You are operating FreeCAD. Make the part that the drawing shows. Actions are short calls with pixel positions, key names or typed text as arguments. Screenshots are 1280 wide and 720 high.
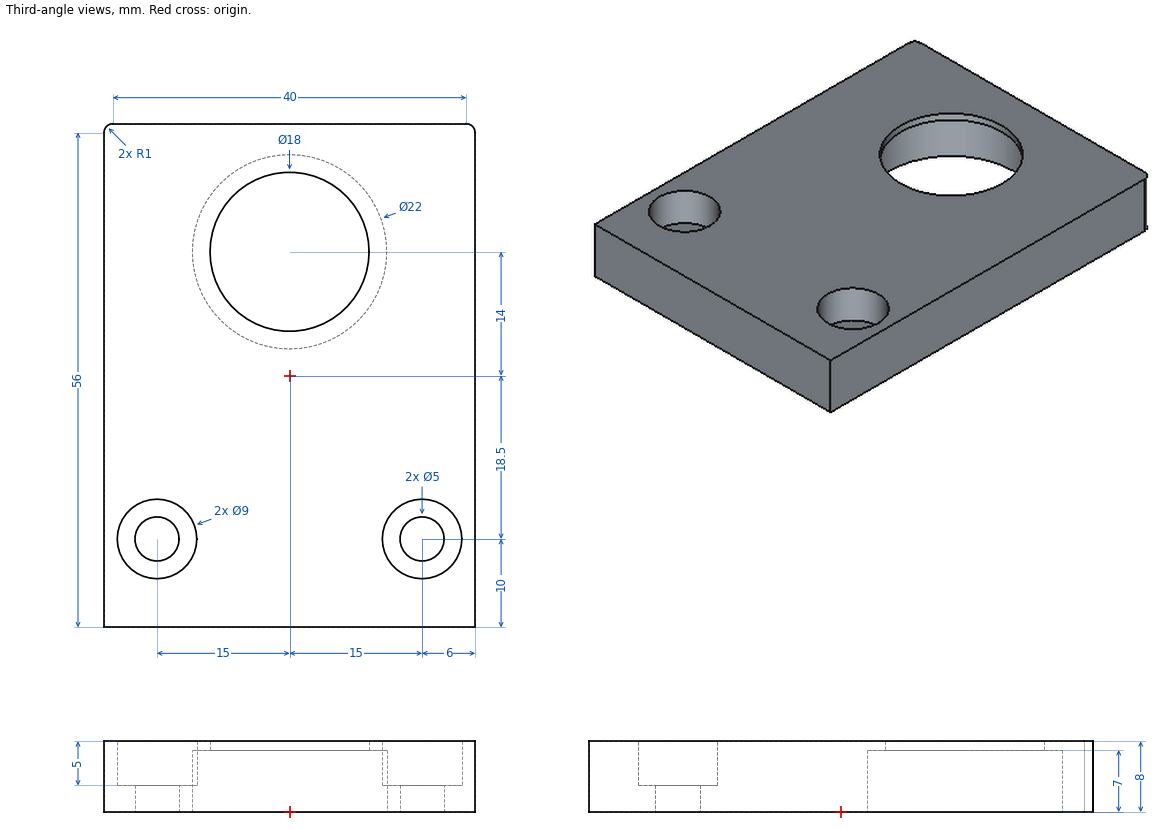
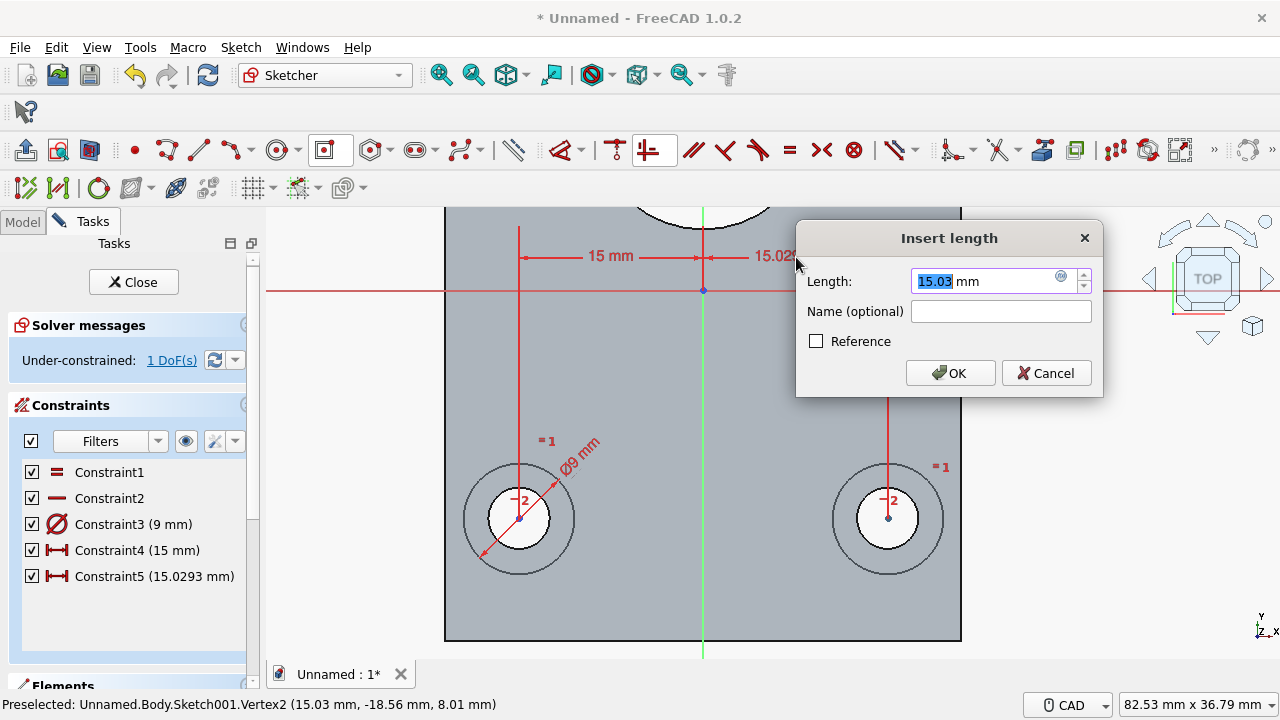
text(15)
key(Return)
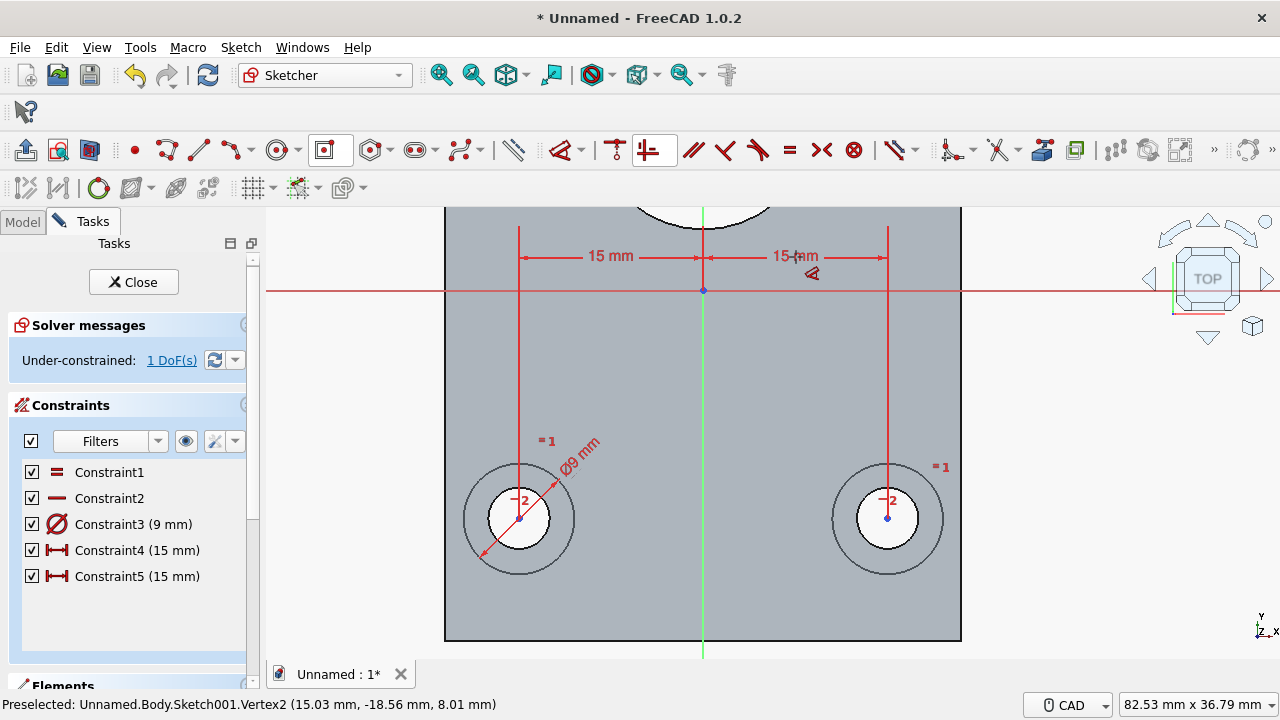
click(519, 519)
click(485, 405)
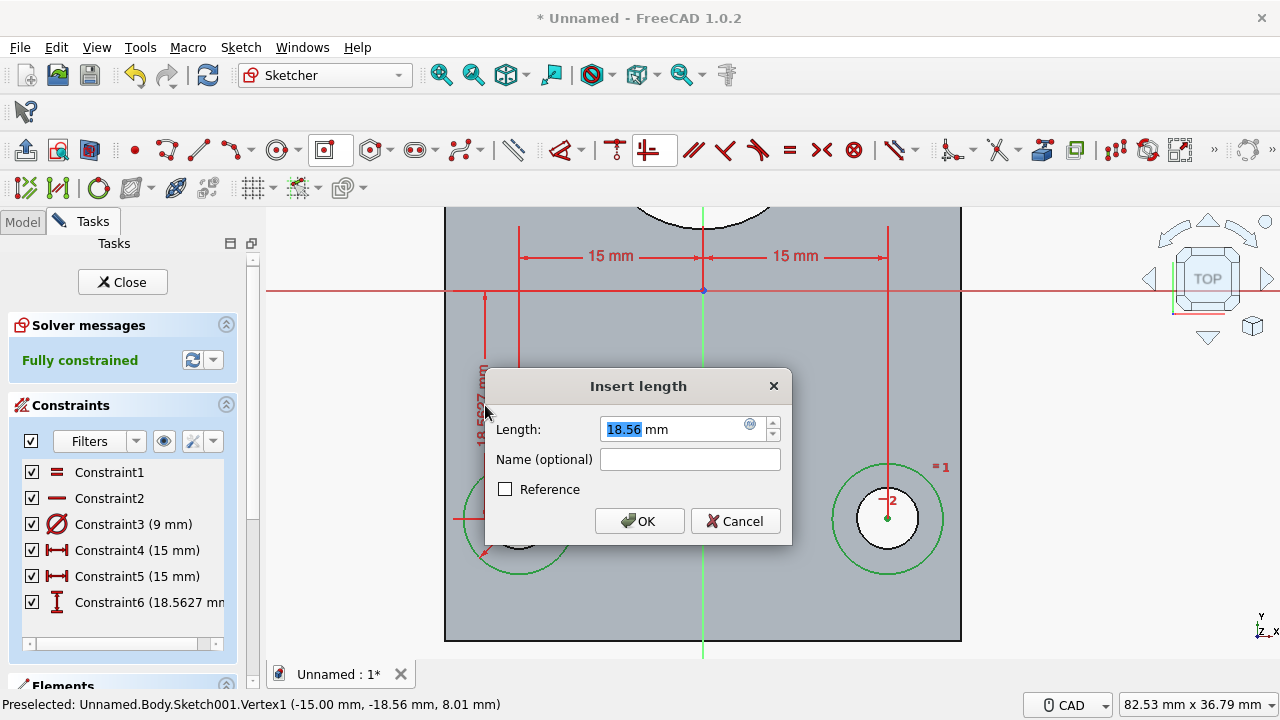
text(18.5)
key(Return)
key(Escape)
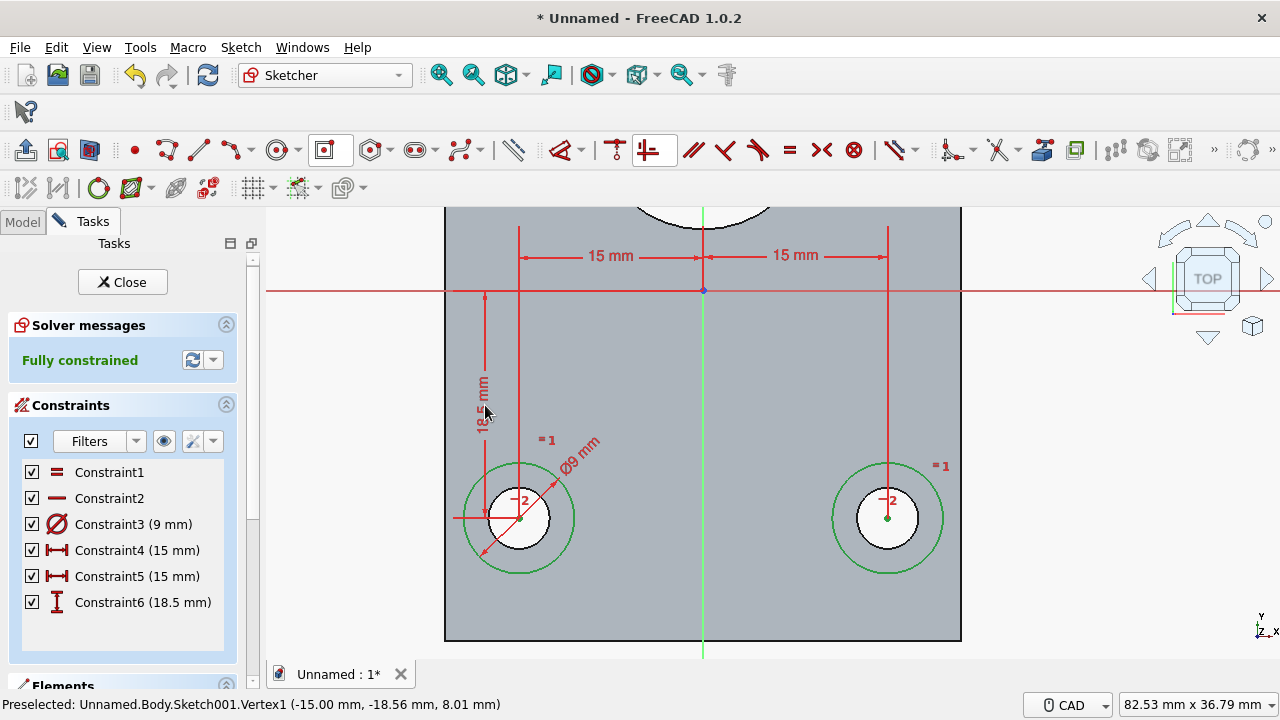
click(123, 282)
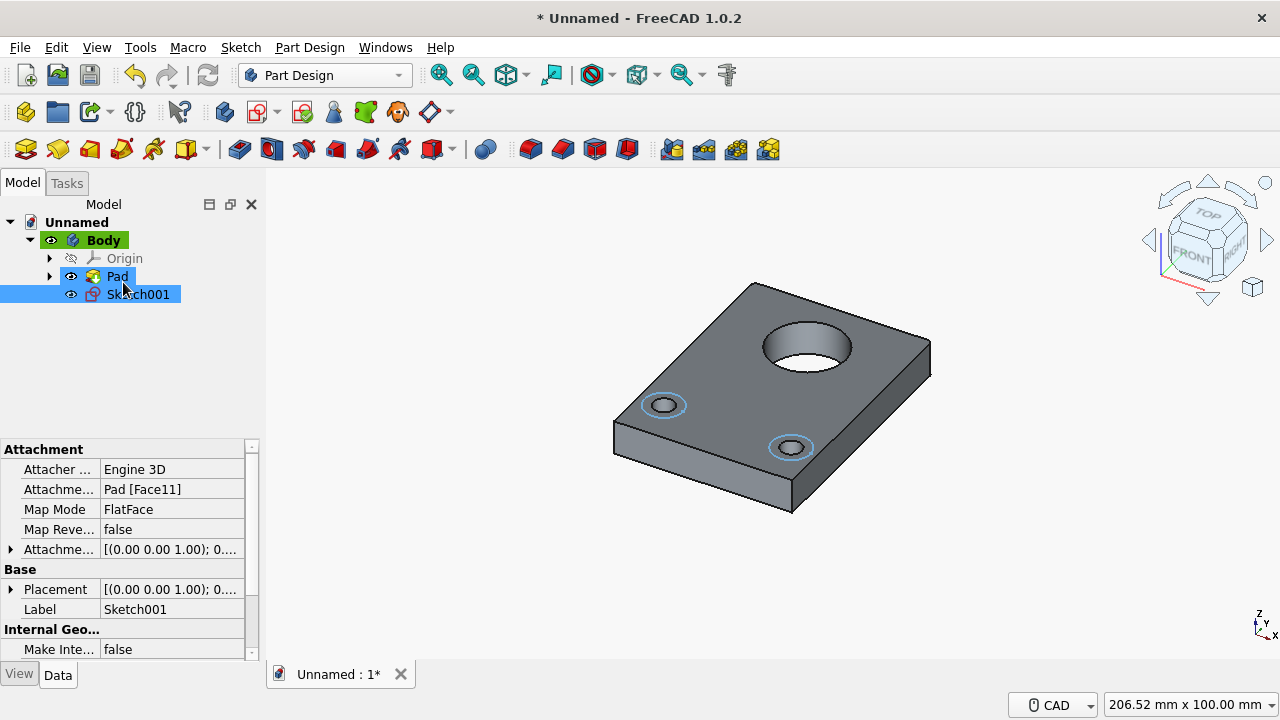
click(240, 150)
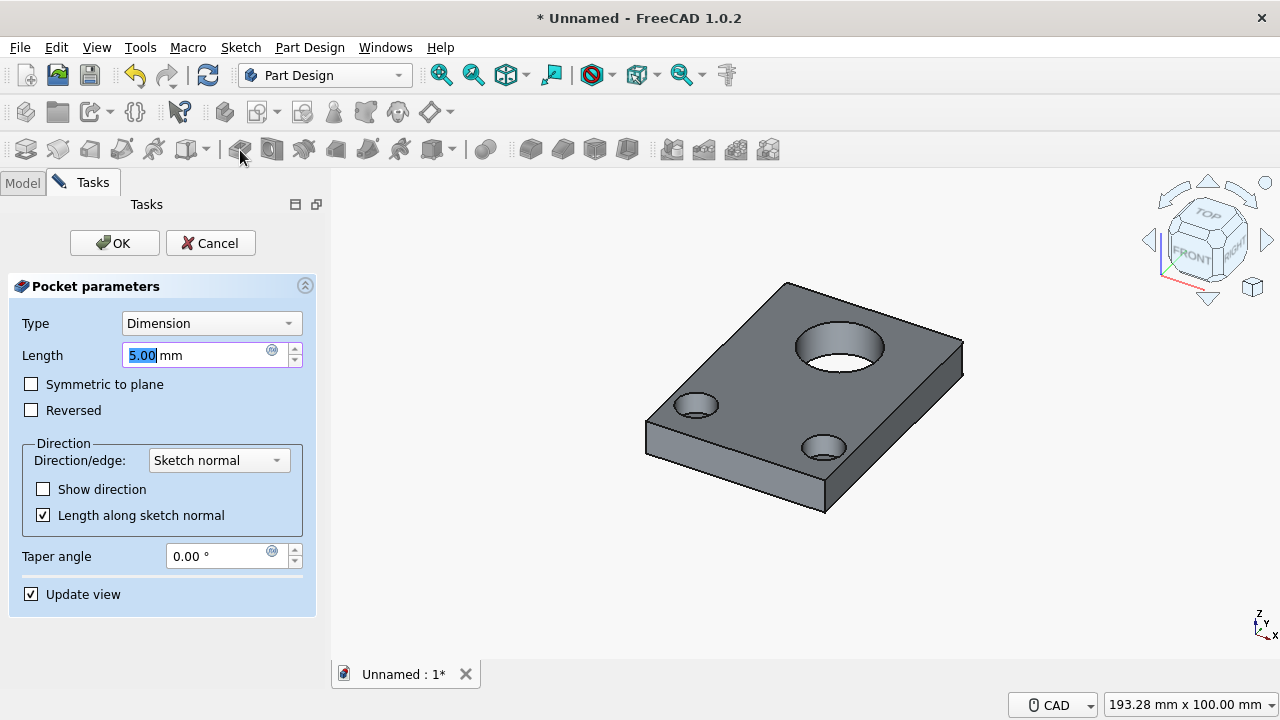
text(5)
key(Tab)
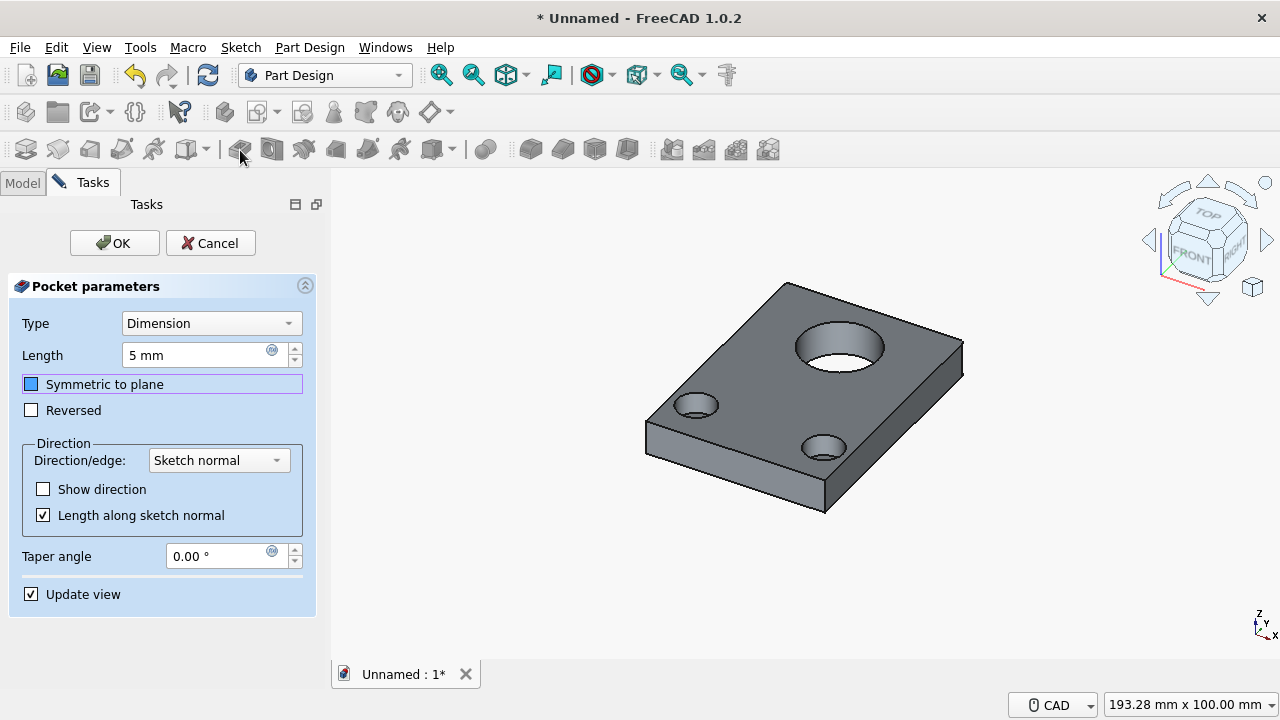
click(115, 243)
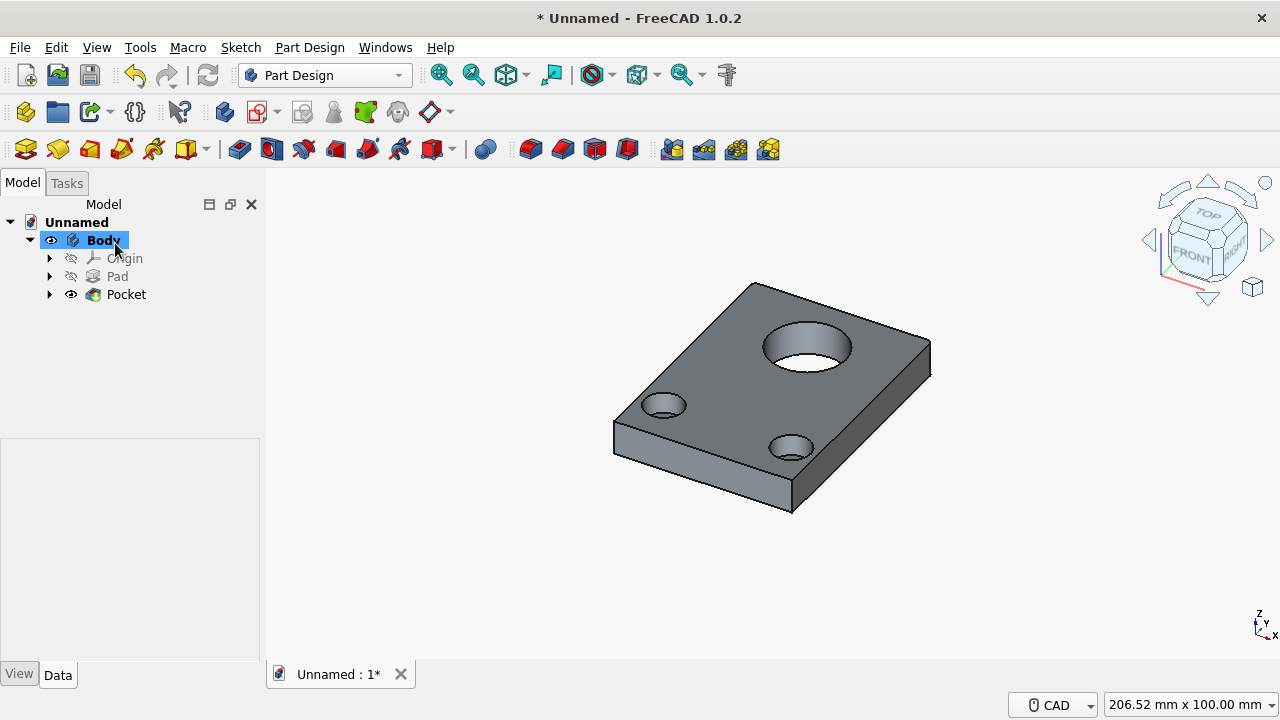
key(5)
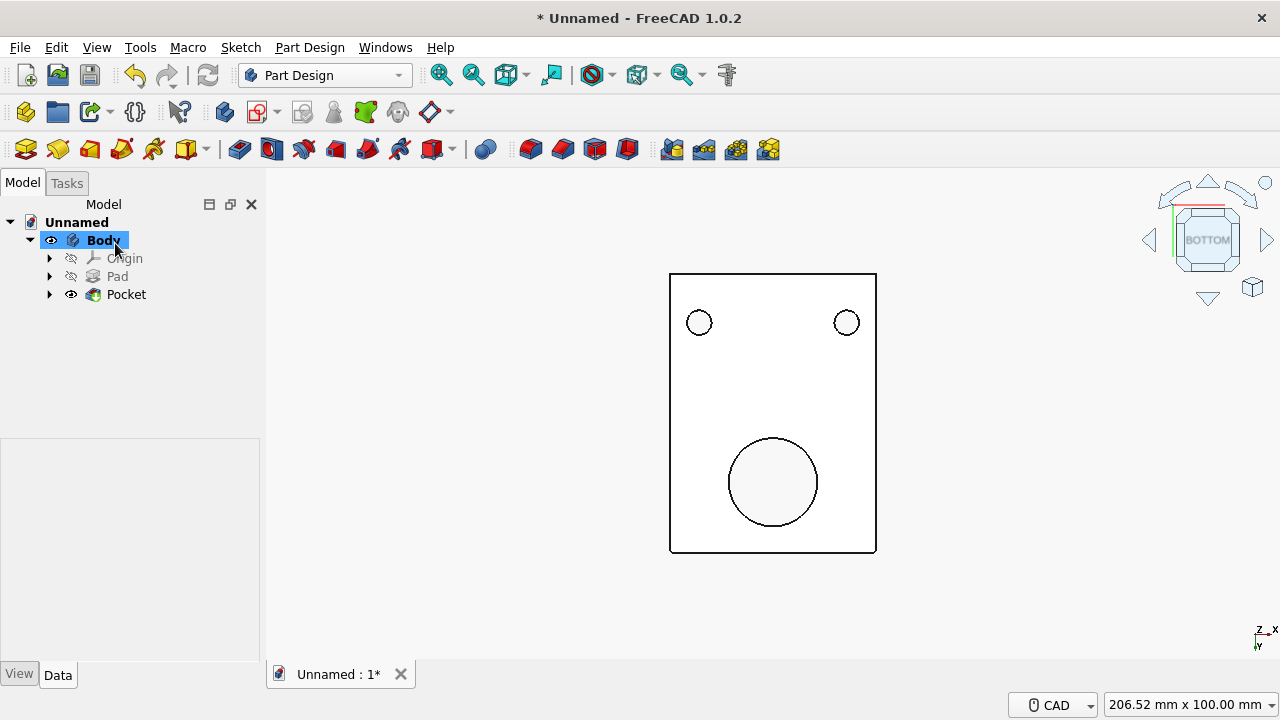
click(773, 373)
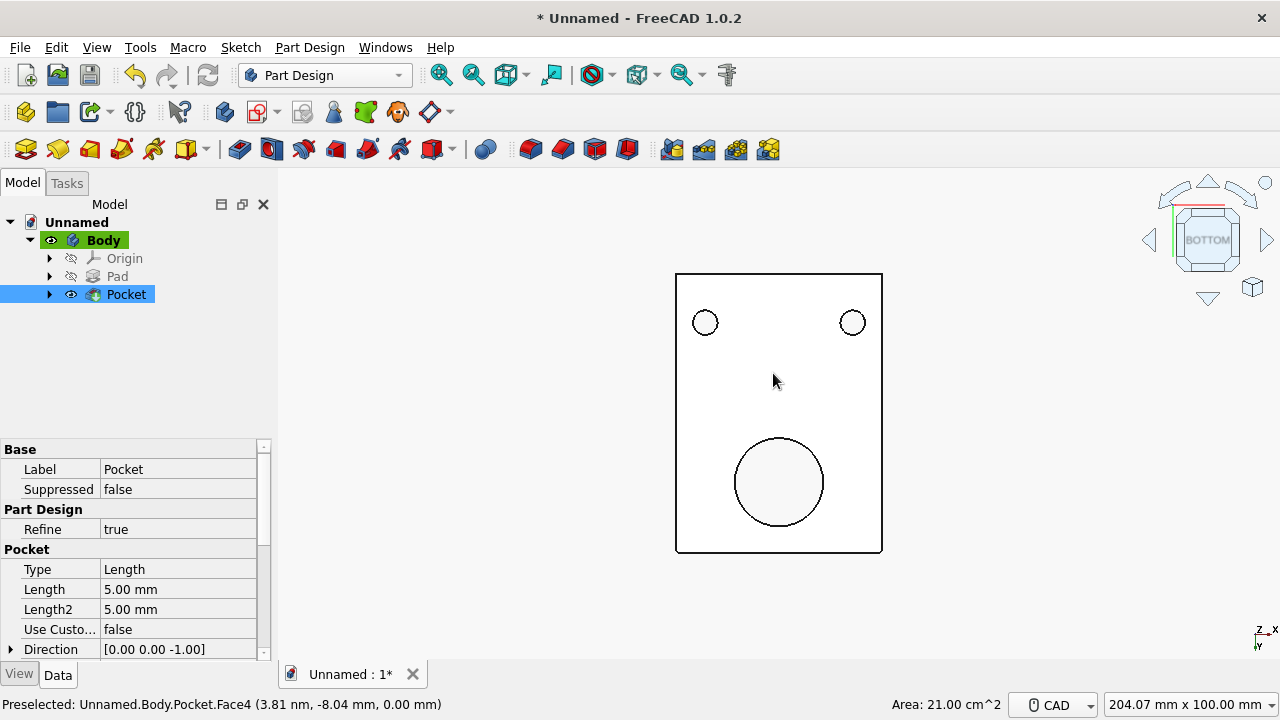
click(258, 112)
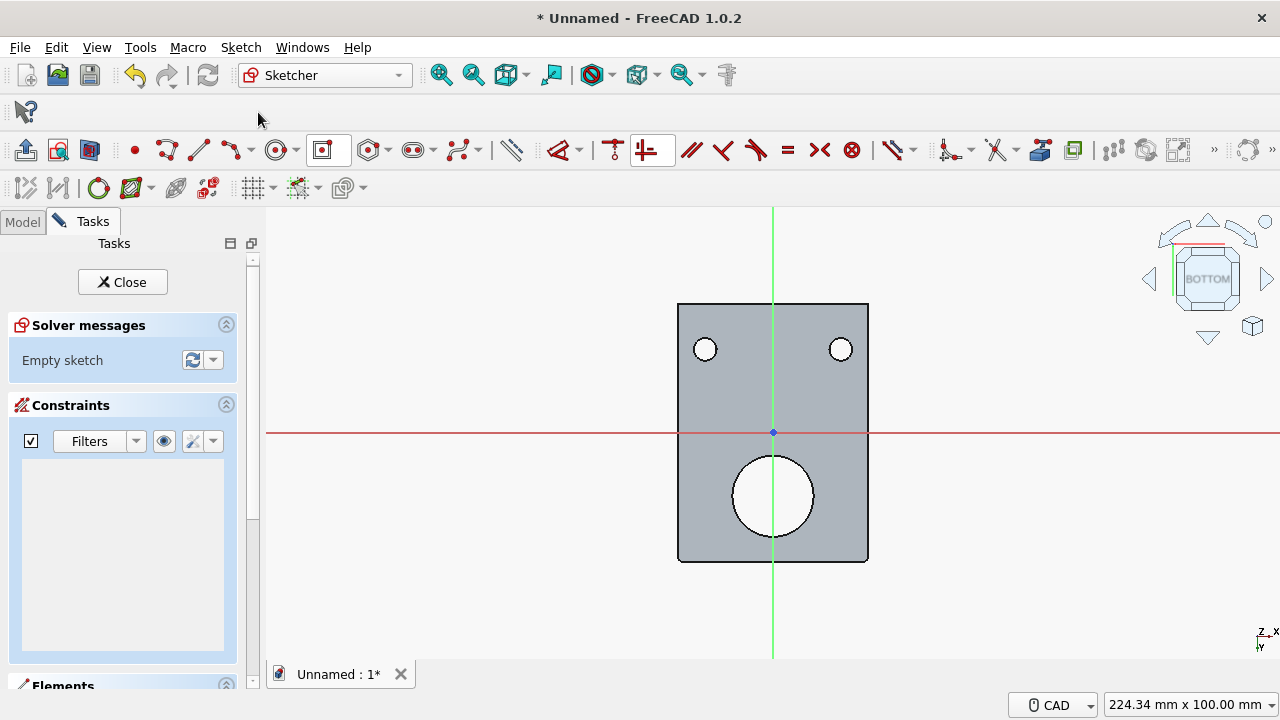
scroll(813, 522, up, 5)